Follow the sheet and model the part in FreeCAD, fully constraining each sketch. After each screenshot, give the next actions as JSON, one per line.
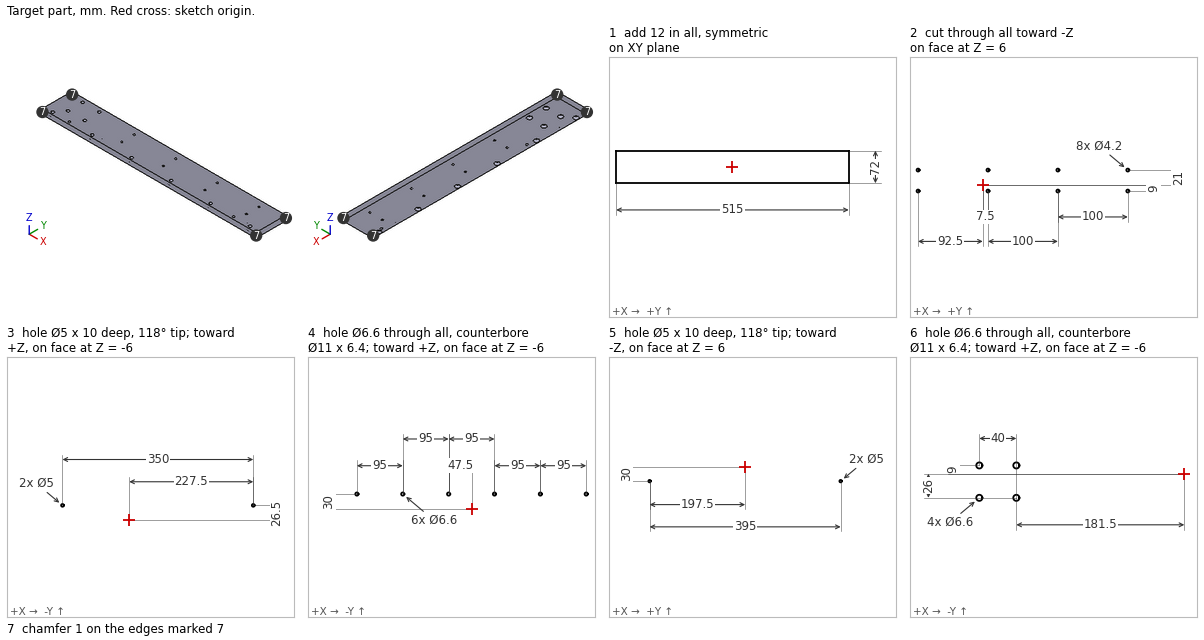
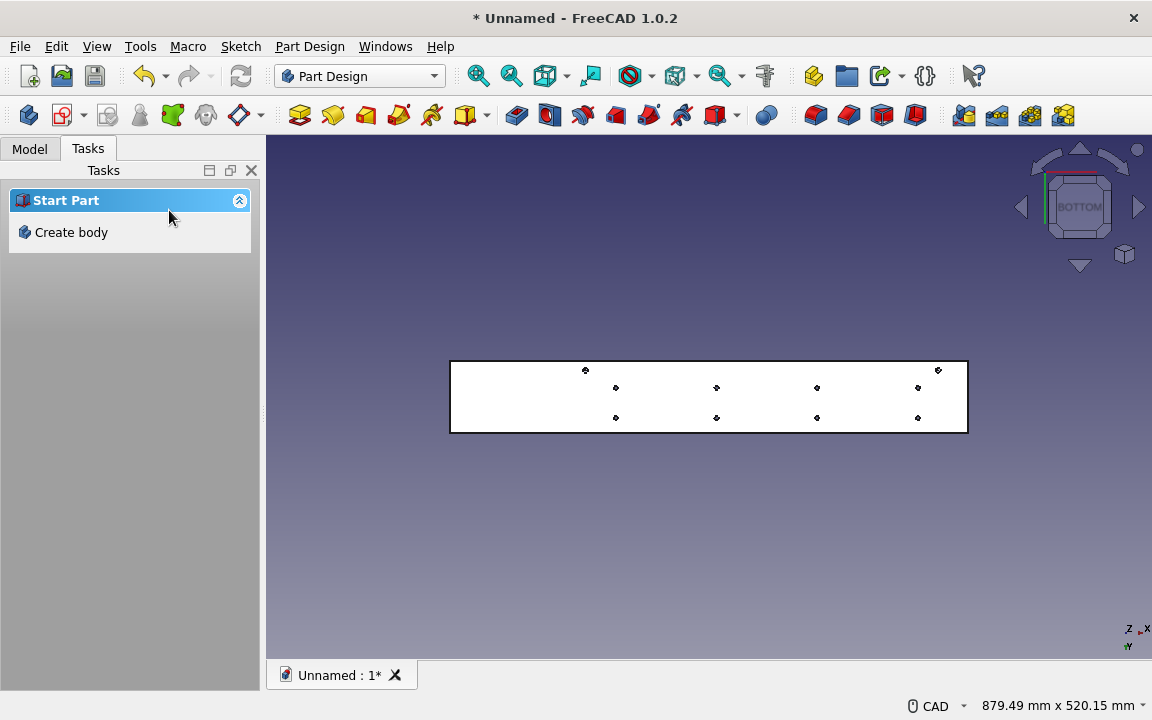
{"action": "left_click", "coordinate": [857, 396]}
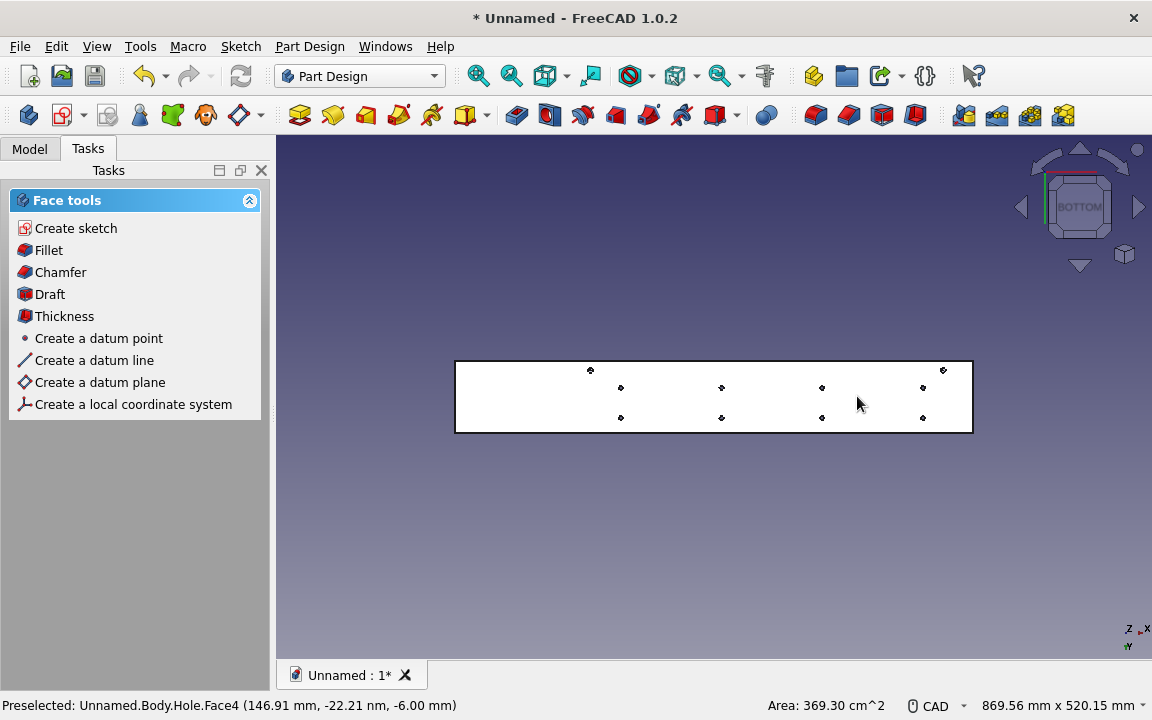
{"action": "left_click", "coordinate": [62, 116]}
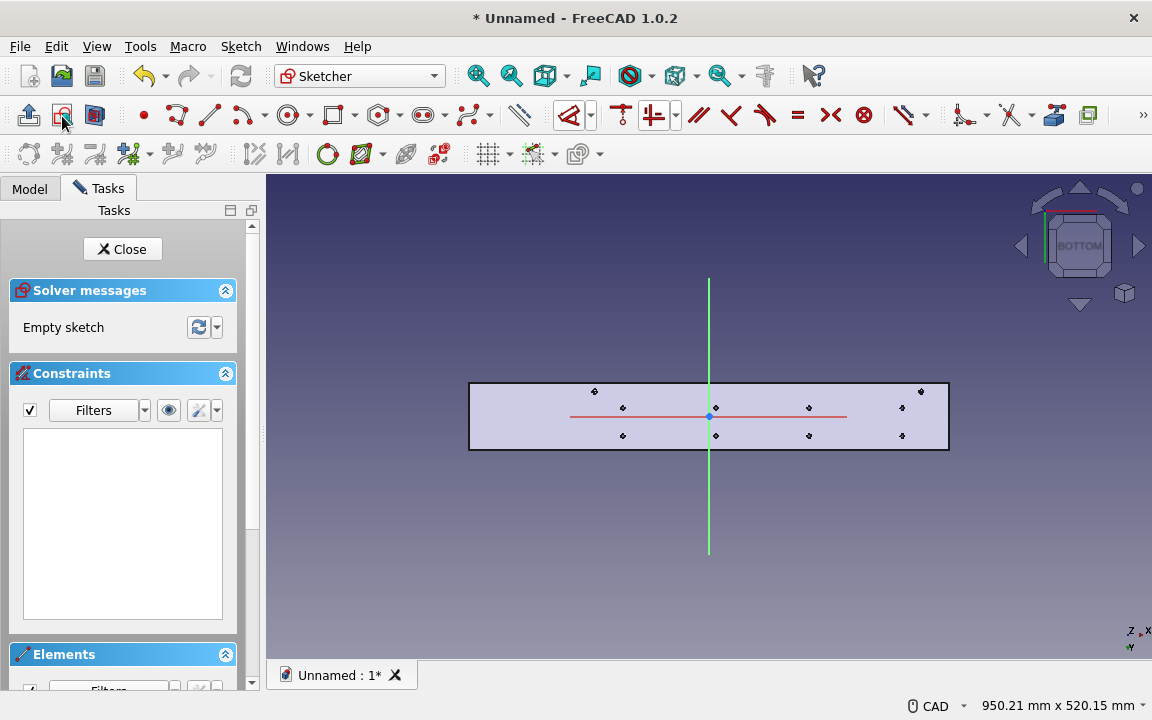
{"action": "left_click", "coordinate": [288, 116]}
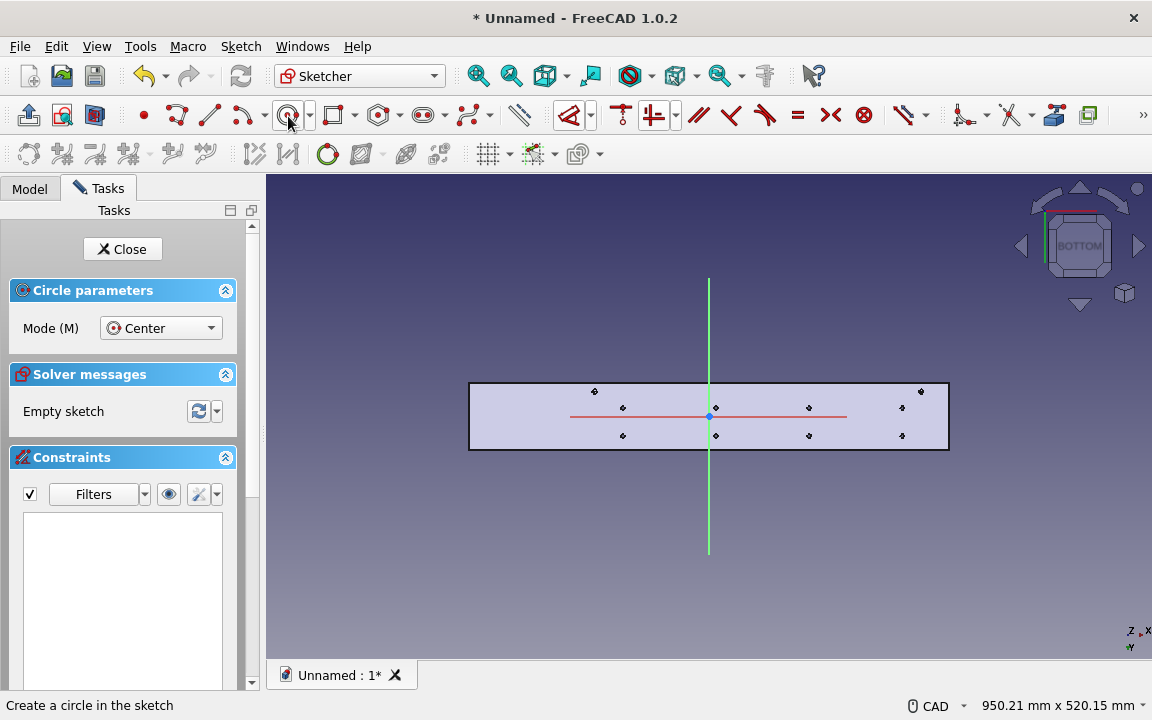
{"action": "scroll", "coordinate": [488, 389], "scroll_direction": "up", "scroll_amount": 10}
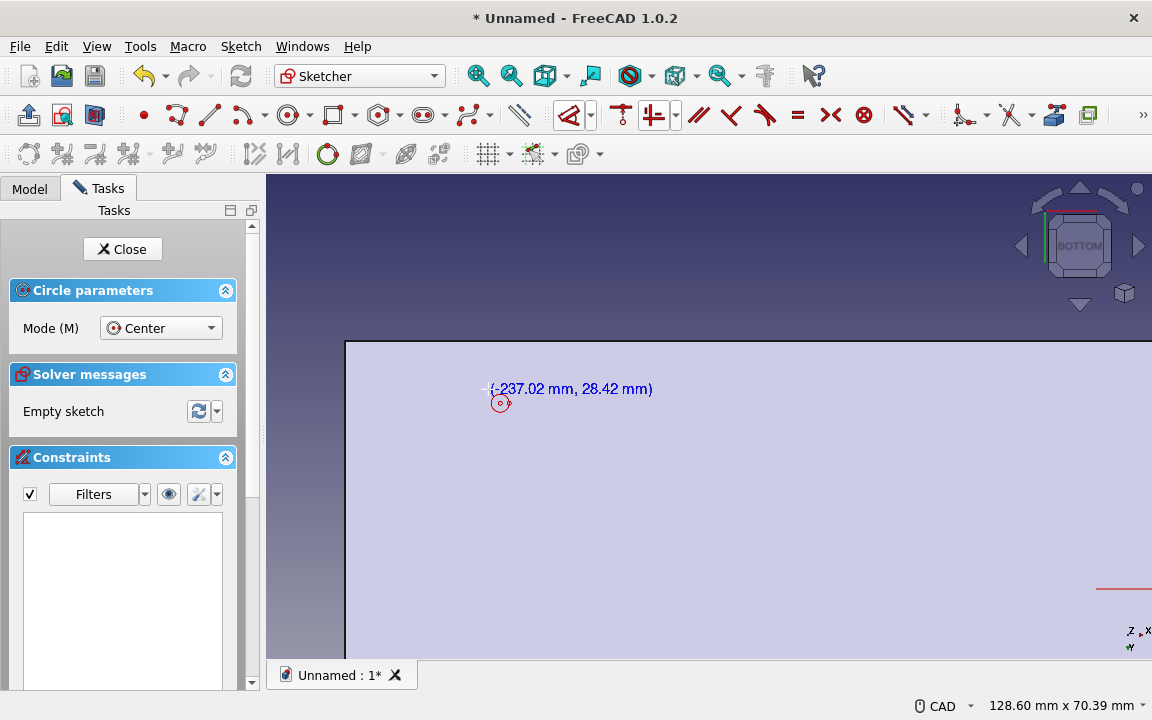
{"action": "scroll", "coordinate": [409, 407], "scroll_direction": "down", "scroll_amount": 10}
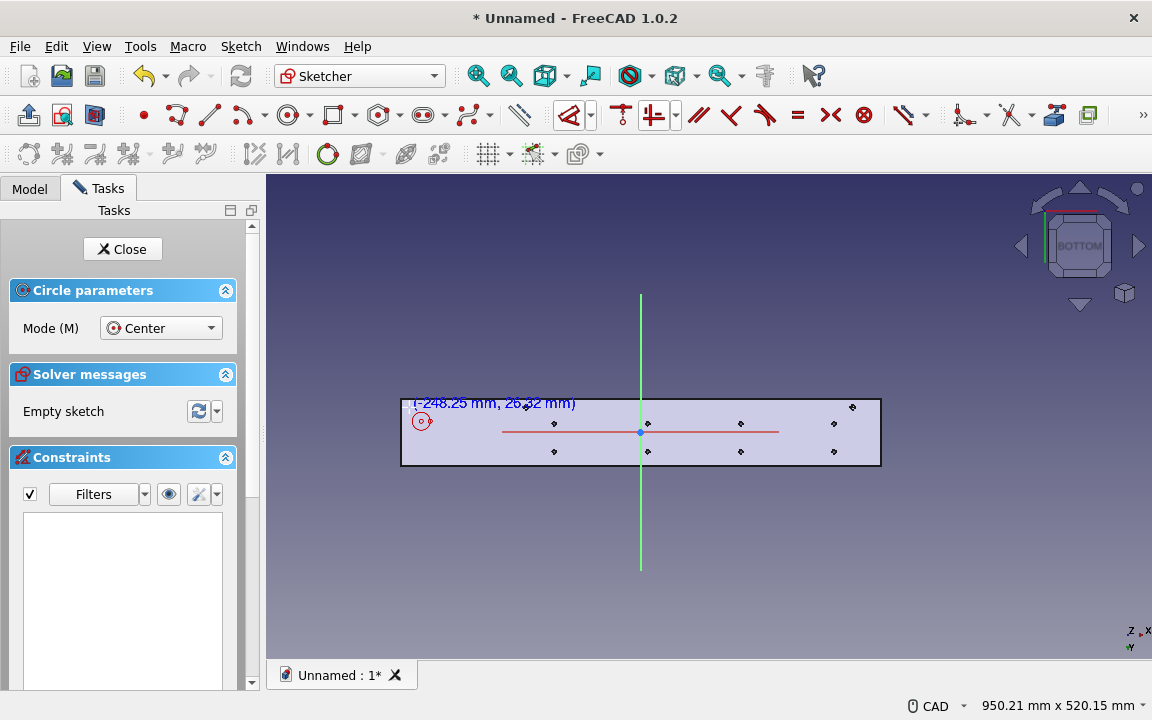
{"action": "left_click", "coordinate": [419, 404]}
{"action": "mouse_move", "coordinate": [421, 402]}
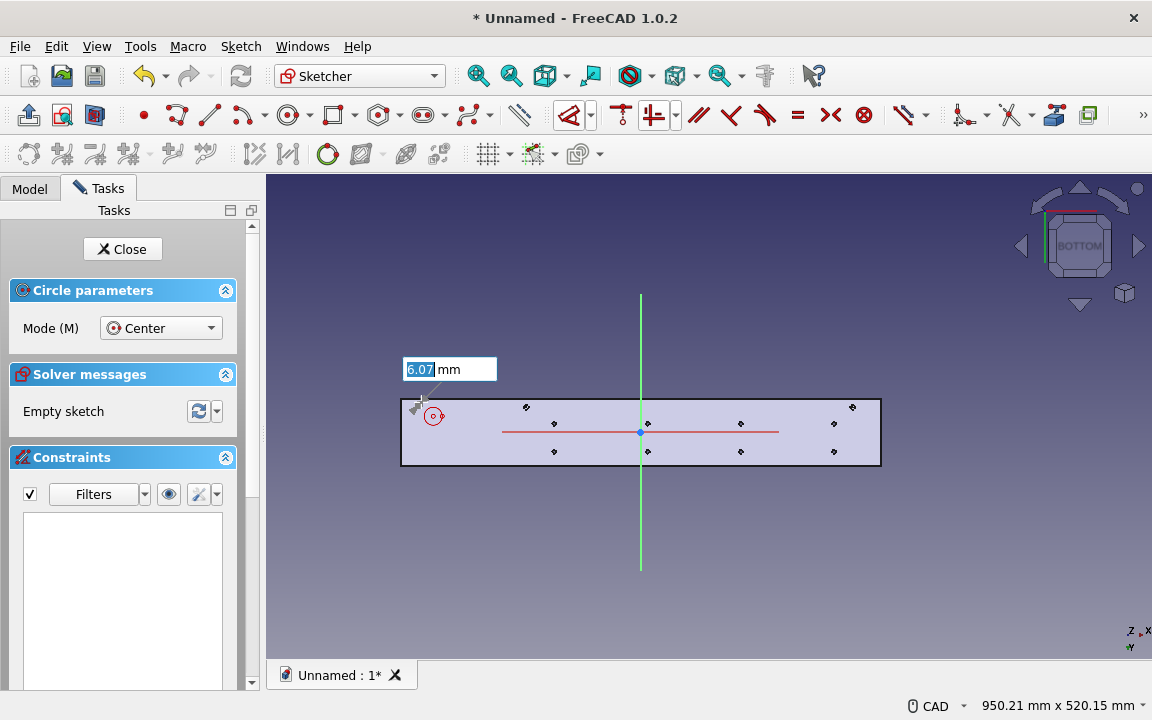
{"action": "type", "text": "6.6"}
{"action": "key", "text": "Return"}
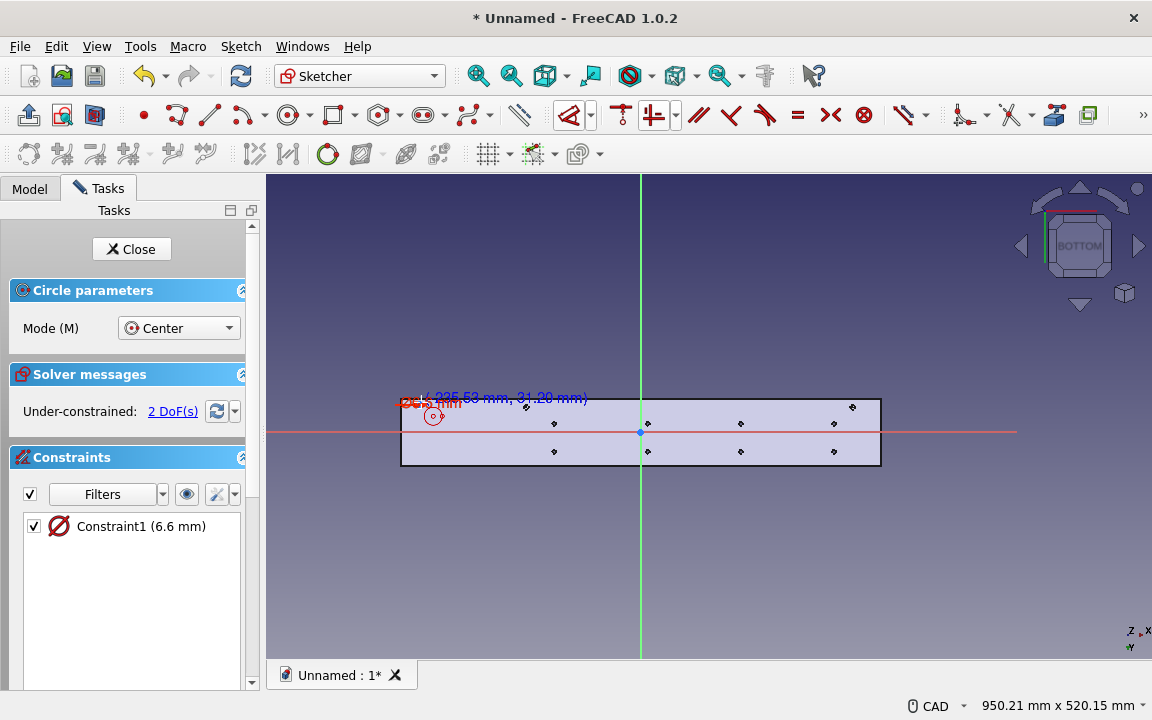
{"action": "scroll", "coordinate": [508, 404], "scroll_direction": "up", "scroll_amount": 10}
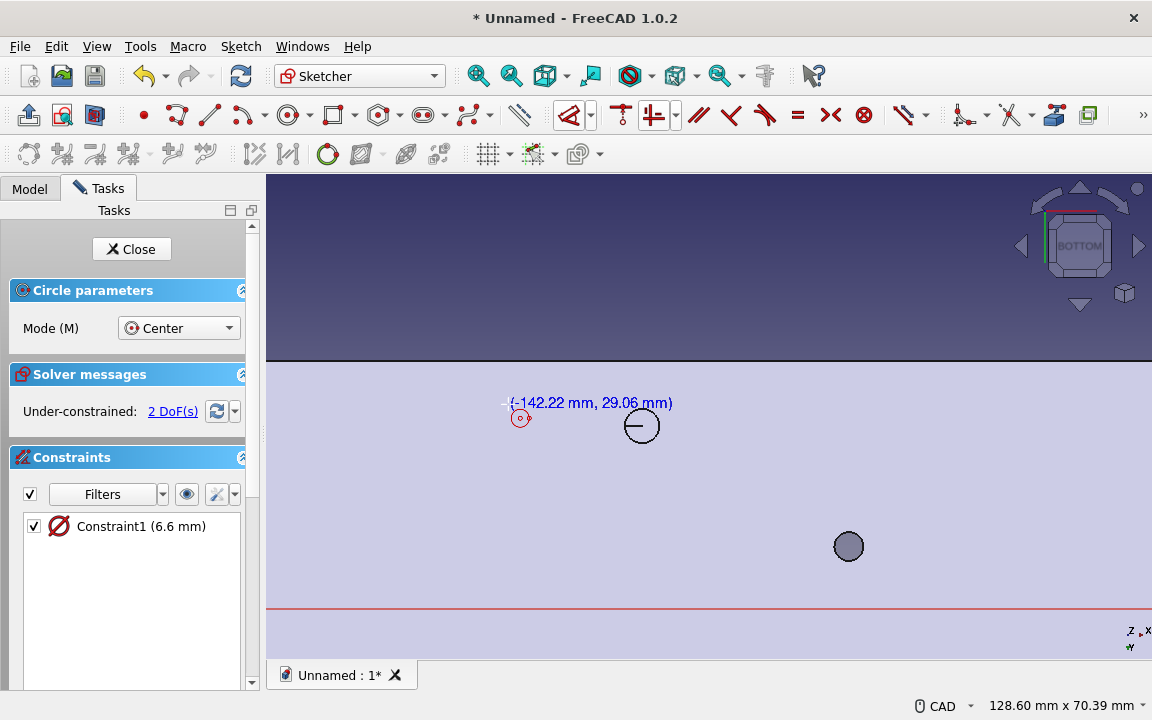
{"action": "scroll", "coordinate": [508, 404], "scroll_direction": "down", "scroll_amount": 10}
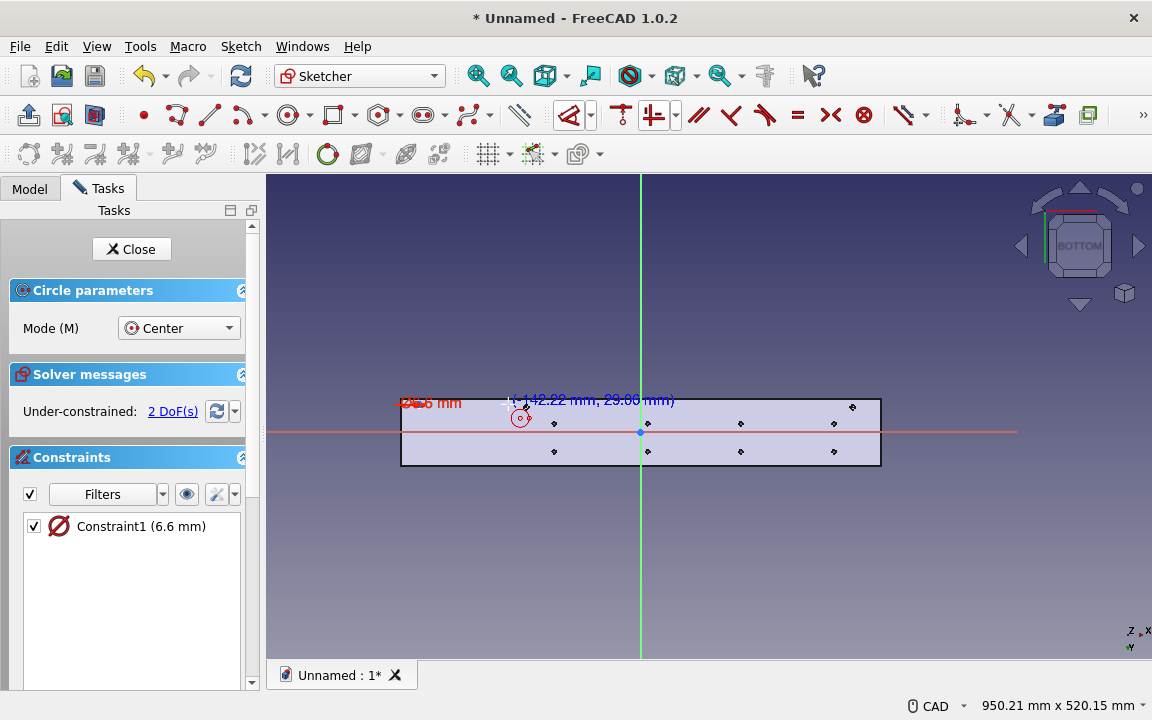
{"action": "left_click", "coordinate": [508, 404]}
{"action": "mouse_move", "coordinate": [510, 402]}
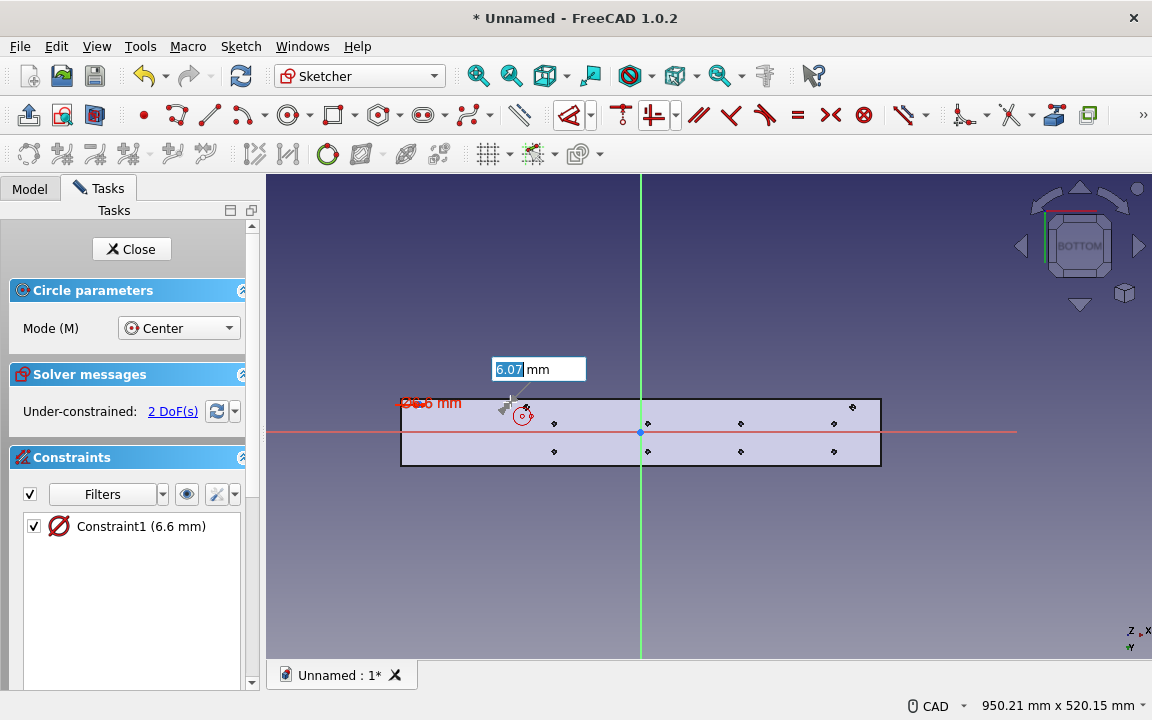
{"action": "type", "text": "6.6"}
{"action": "key", "text": "Return"}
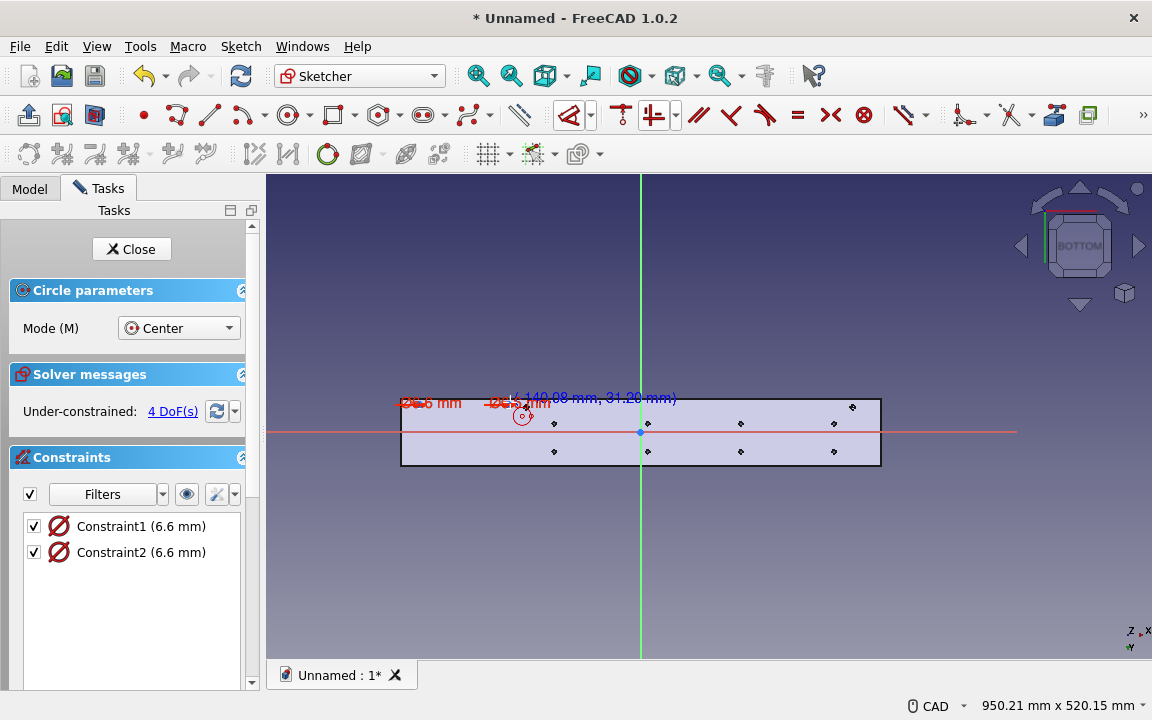
{"action": "scroll", "coordinate": [596, 404], "scroll_direction": "up", "scroll_amount": 10}